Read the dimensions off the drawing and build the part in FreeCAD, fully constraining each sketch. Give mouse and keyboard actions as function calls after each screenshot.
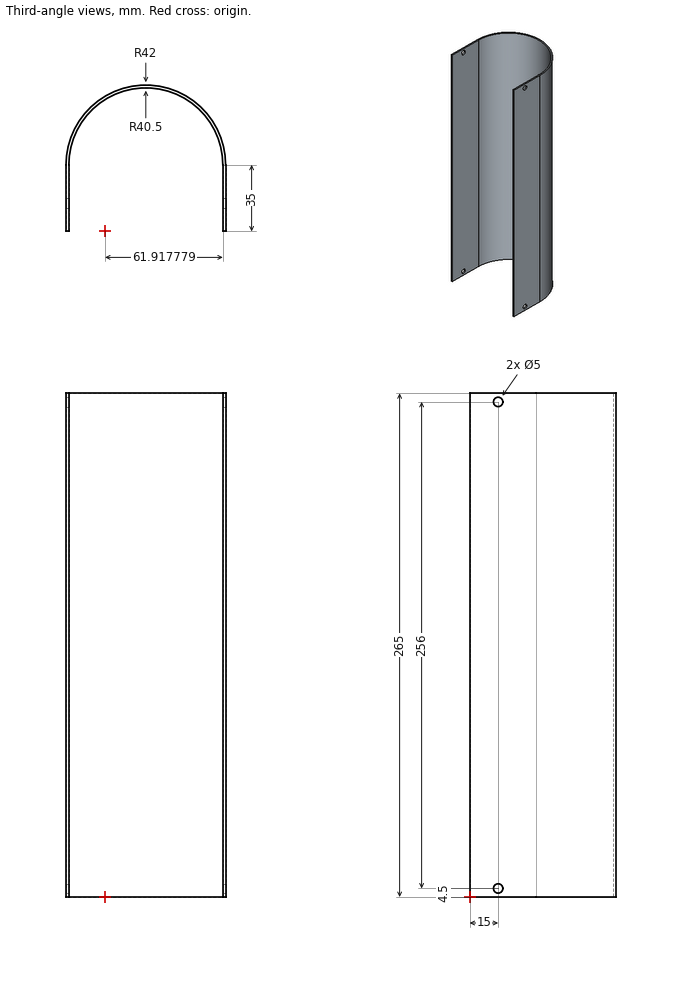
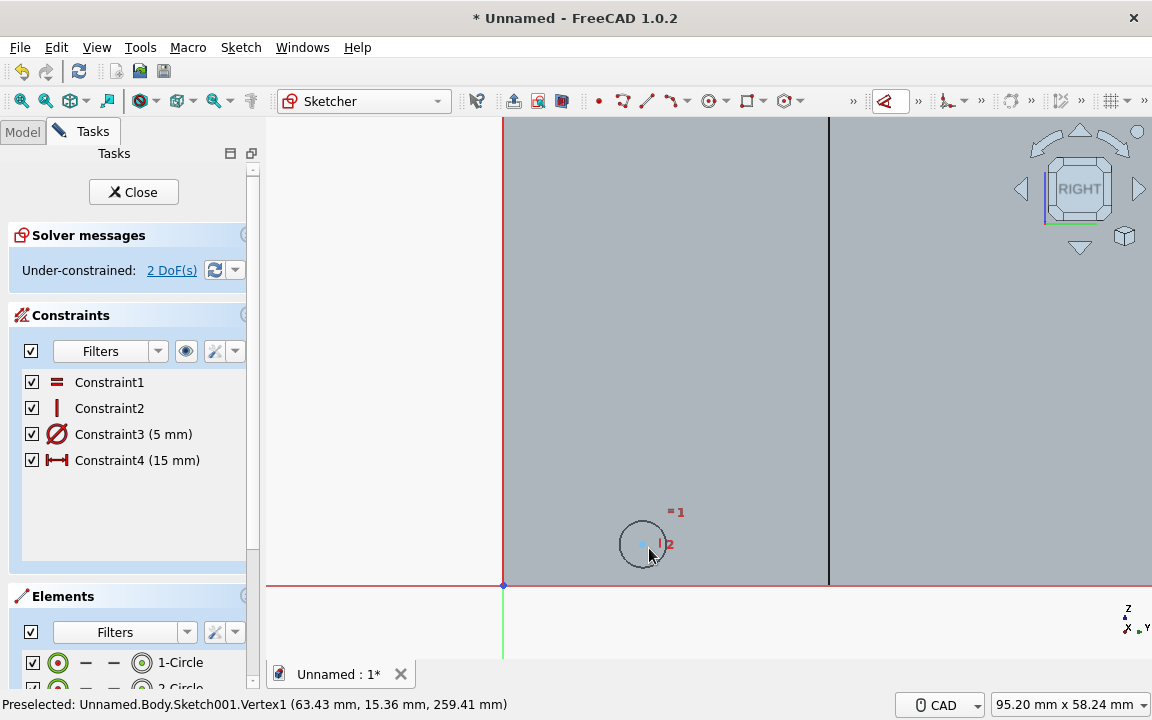
click(643, 544)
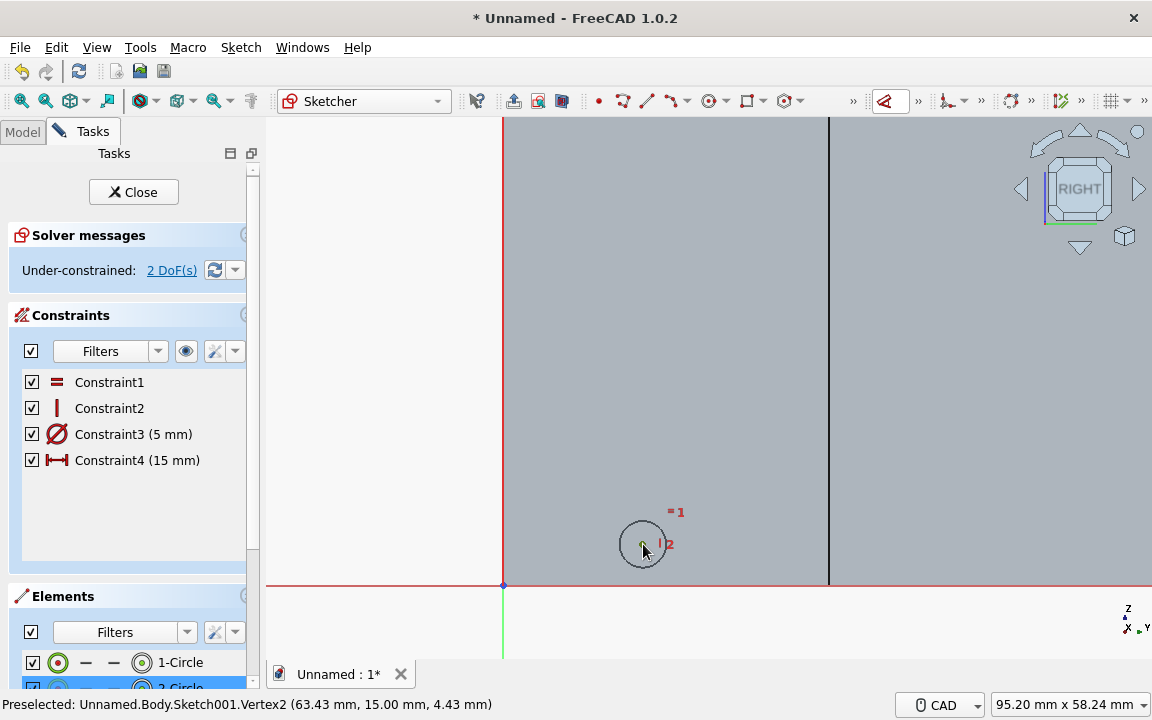
click(904, 102)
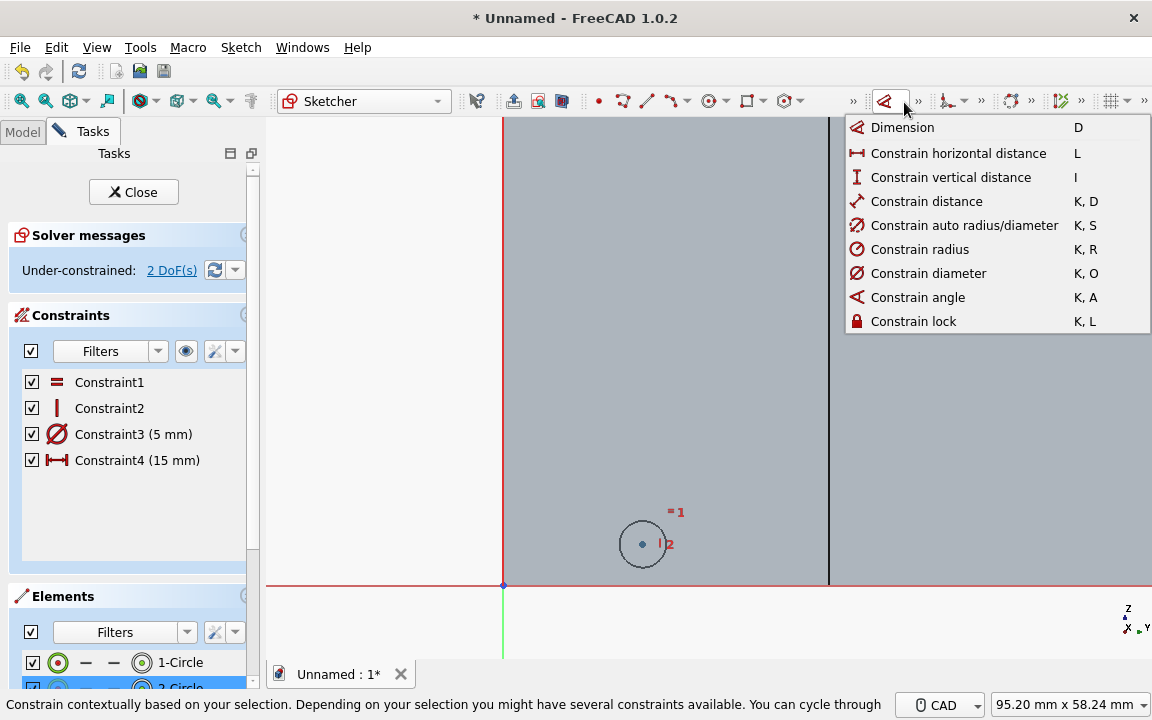
click(998, 177)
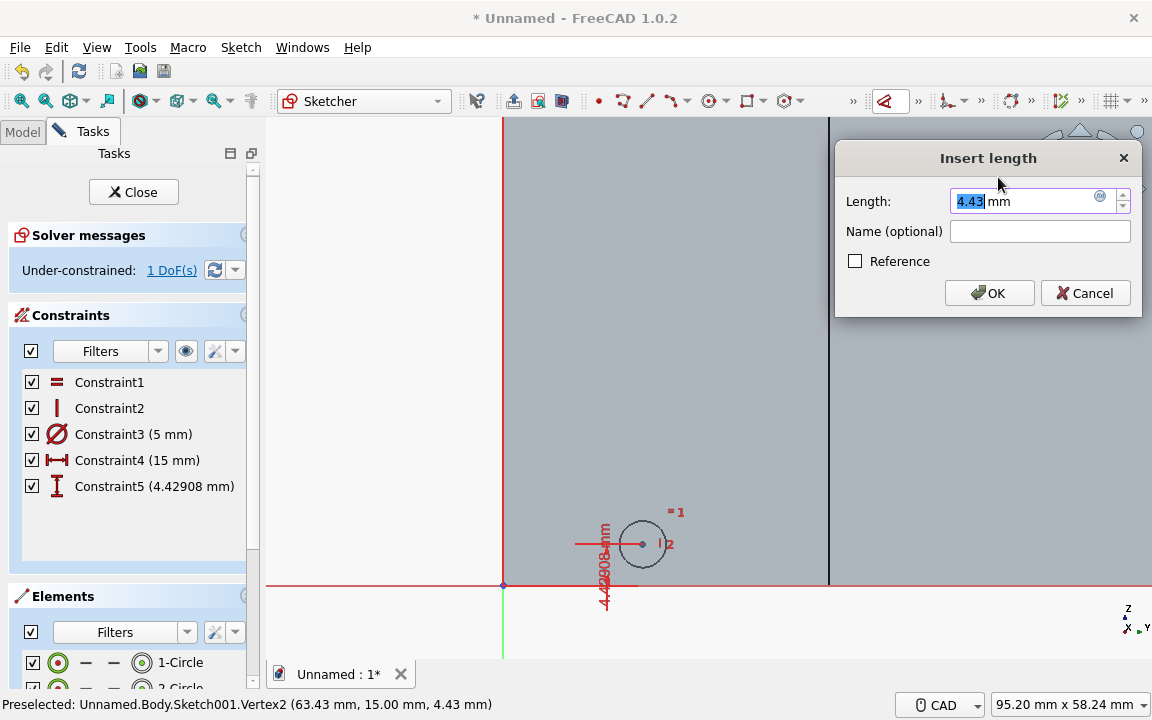
text(4.5)
key(Return)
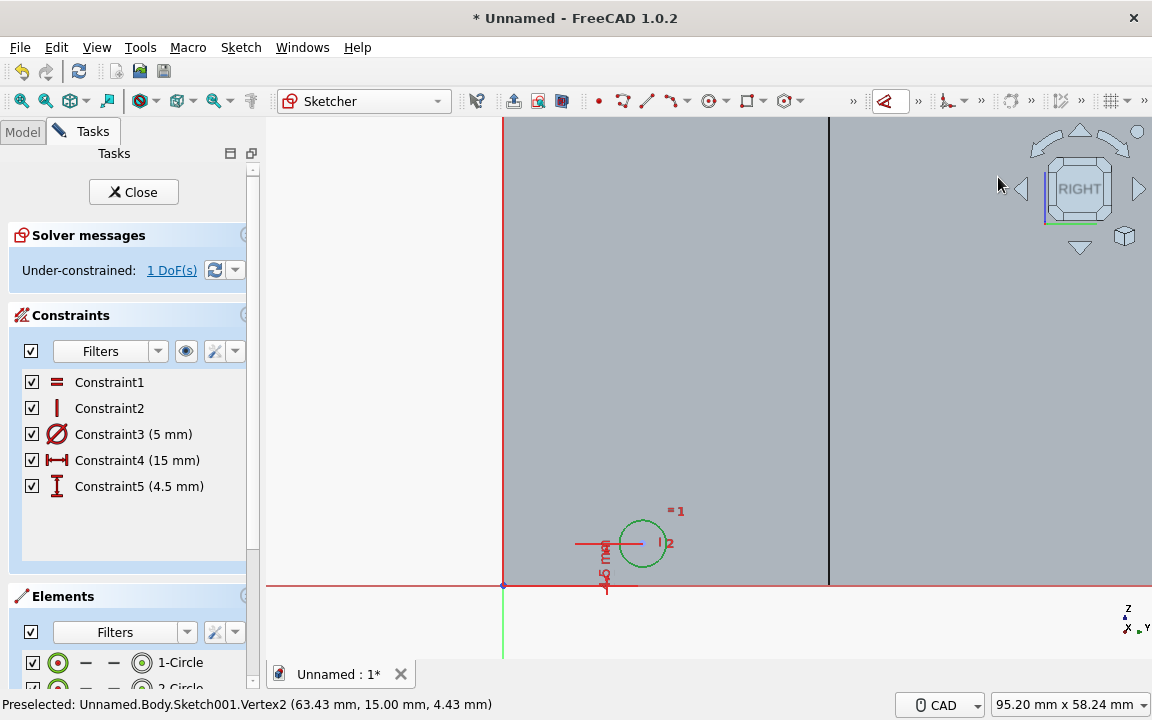
scroll(649, 549, down, 10)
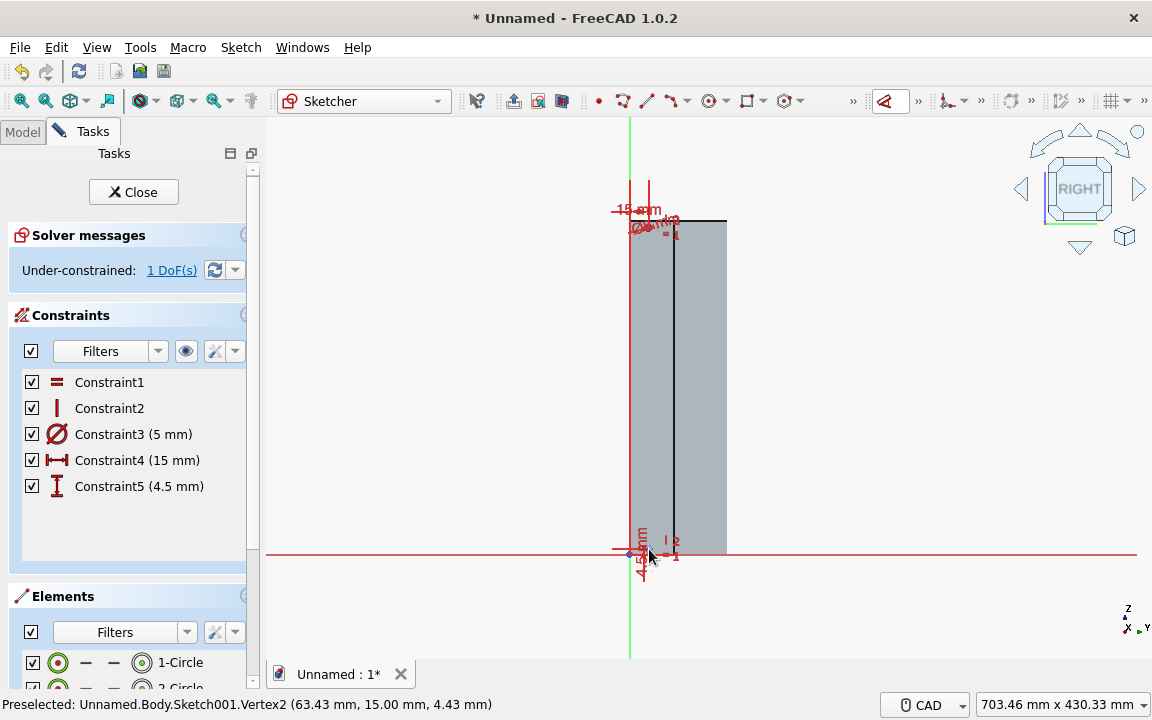
click(649, 228)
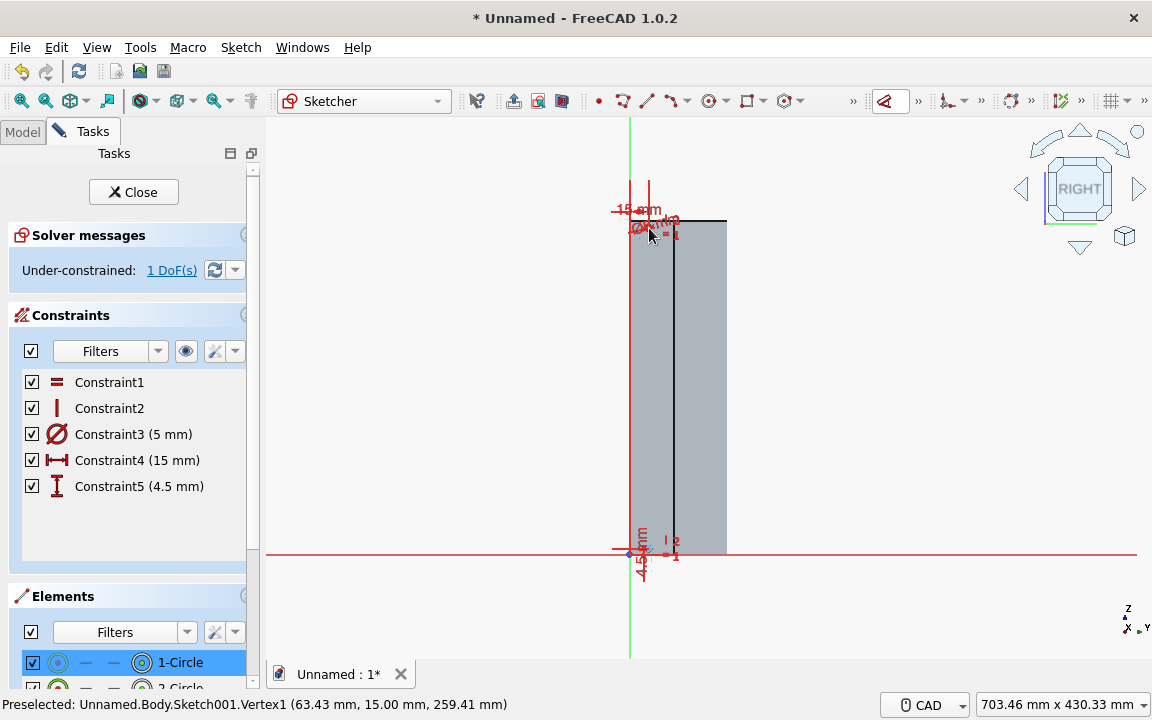
click(649, 549)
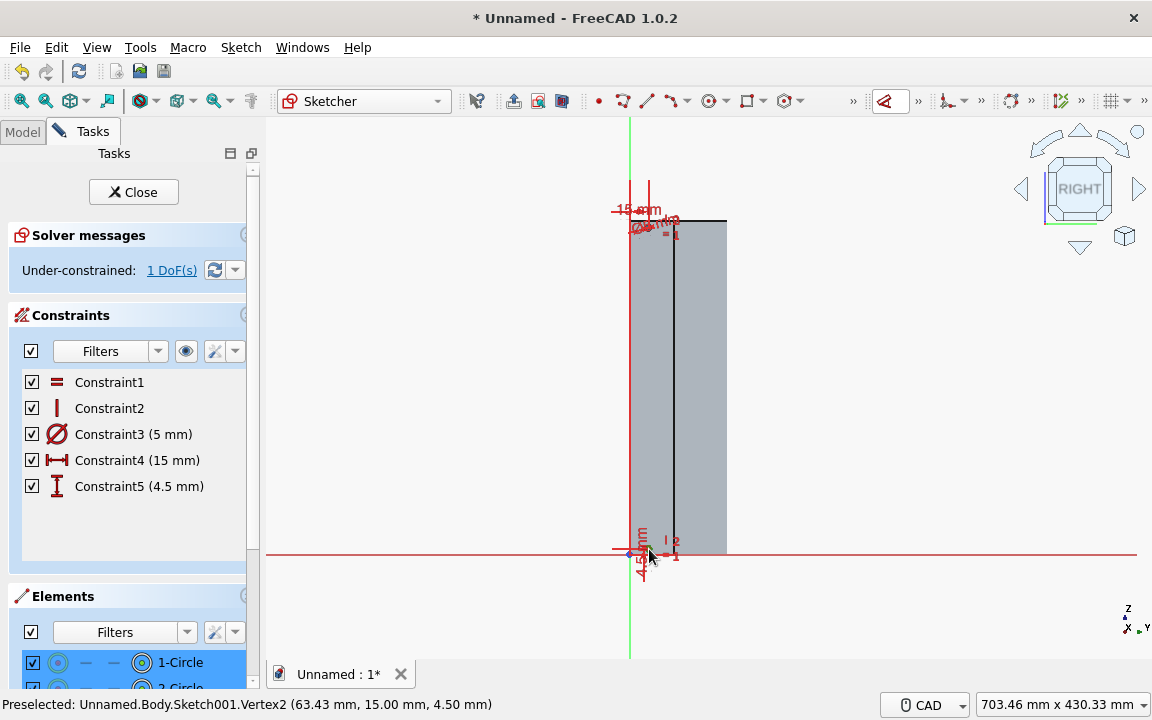
key(i)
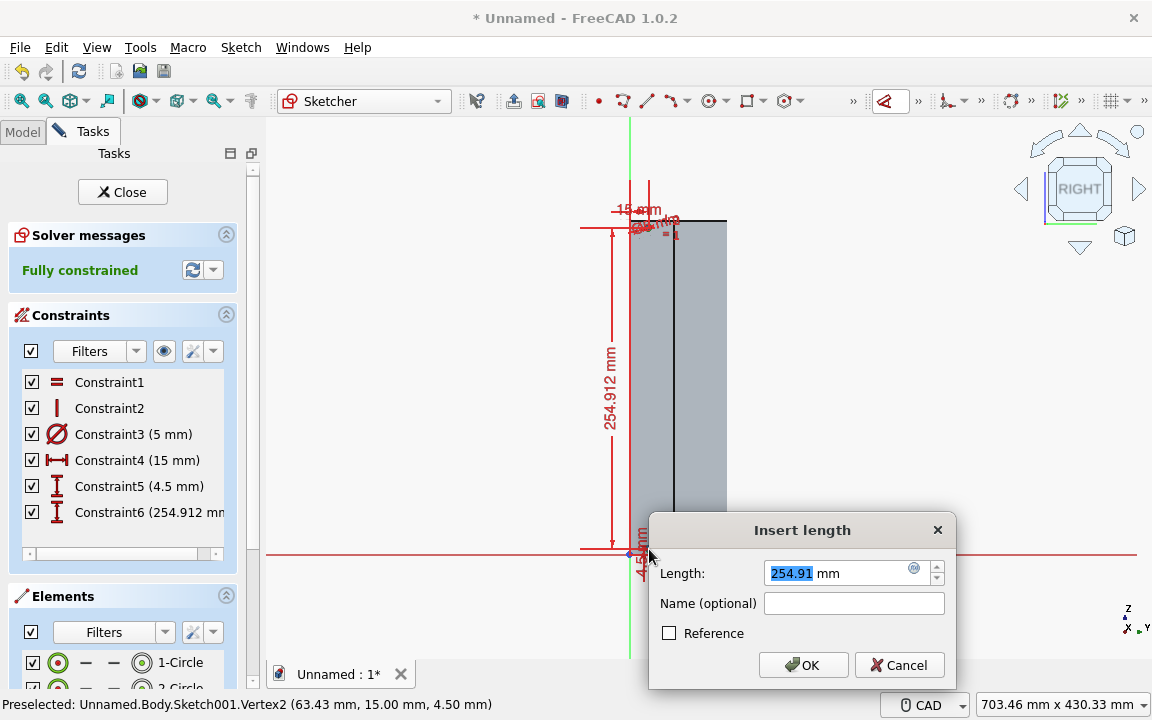
text(256)
key(Return)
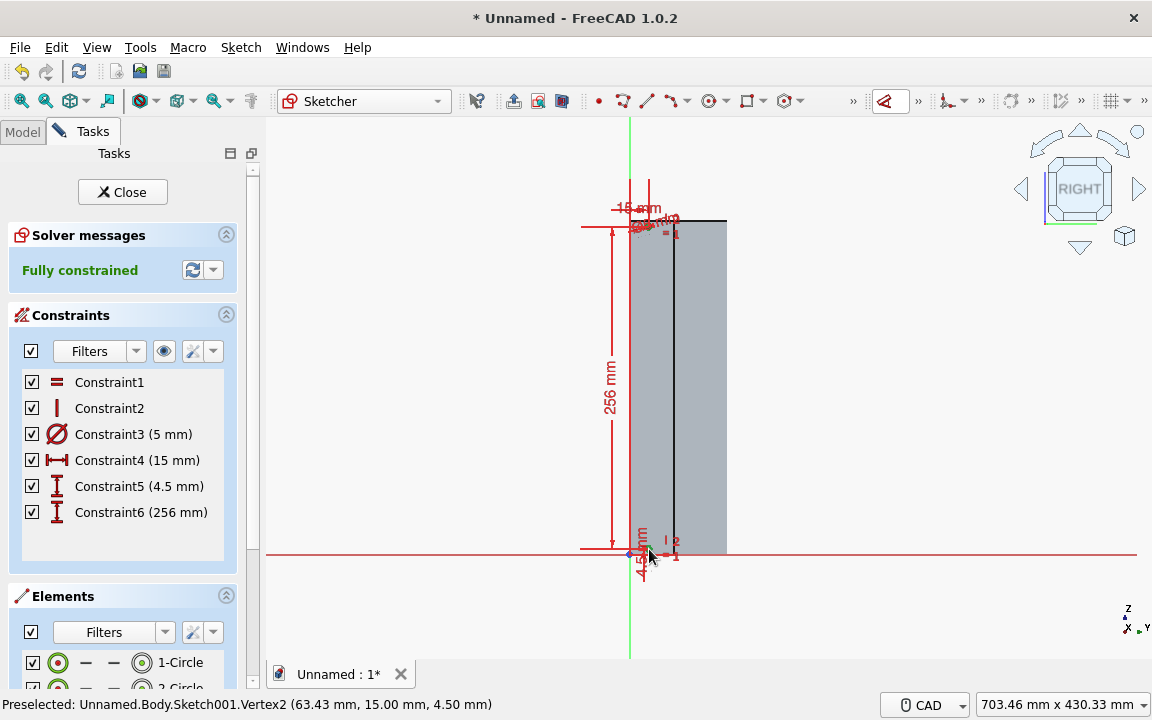
click(123, 192)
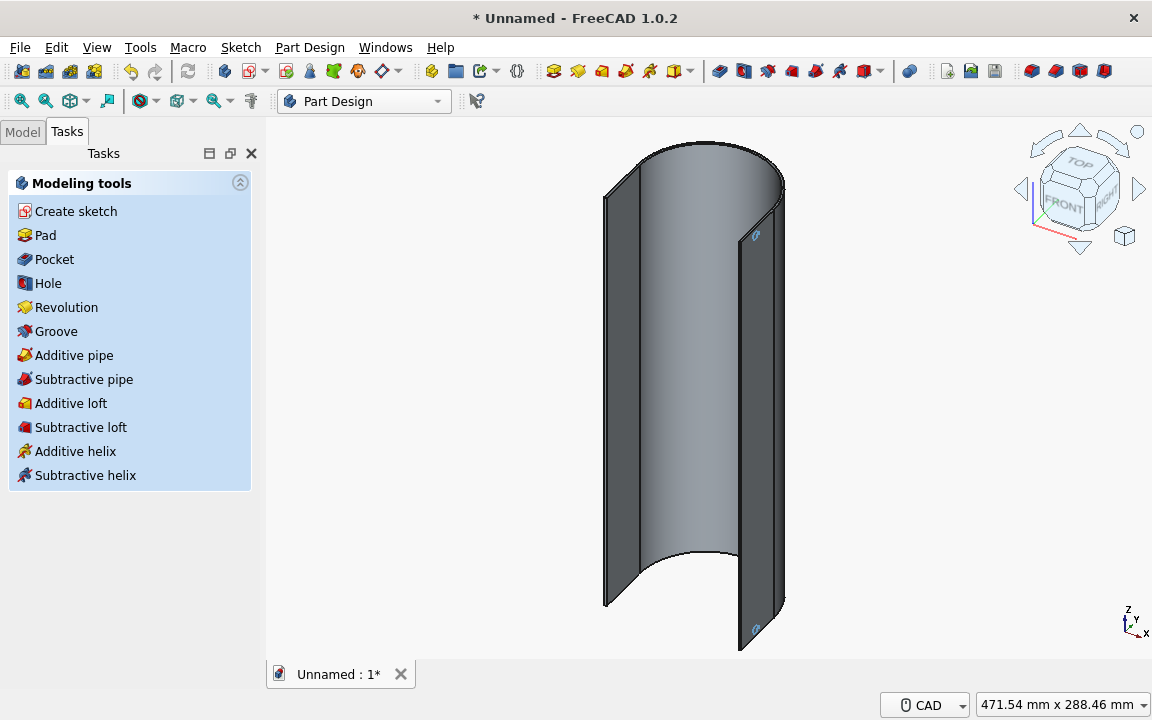
click(720, 72)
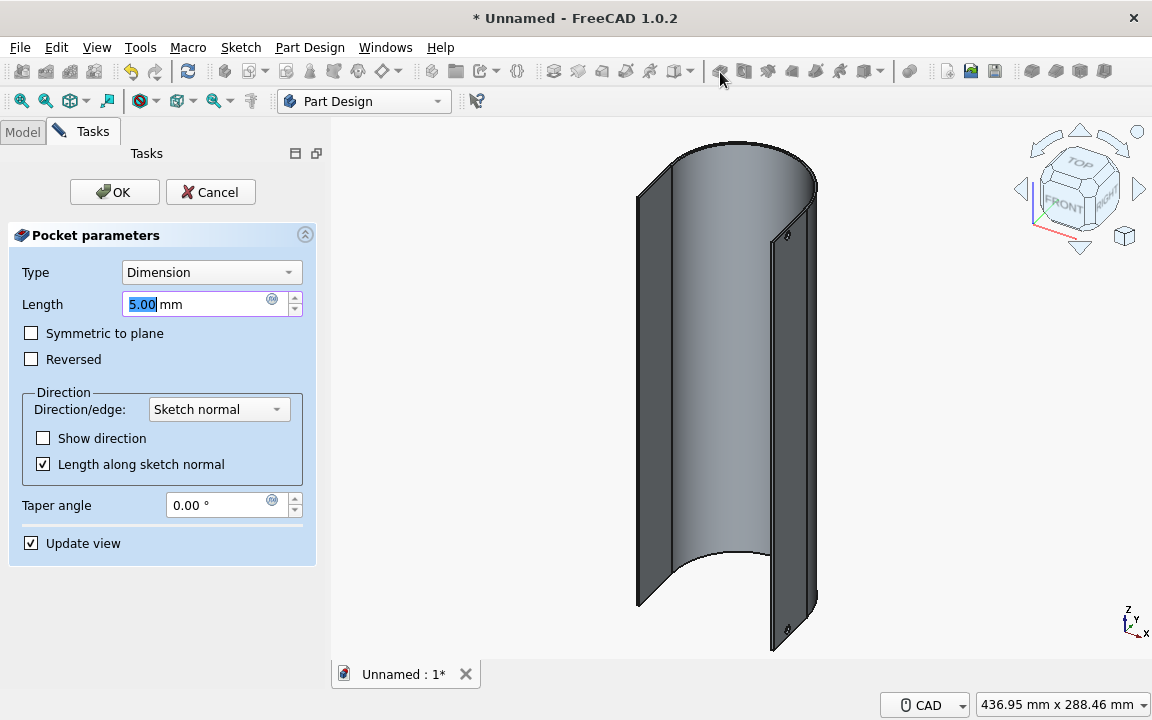
click(212, 272)